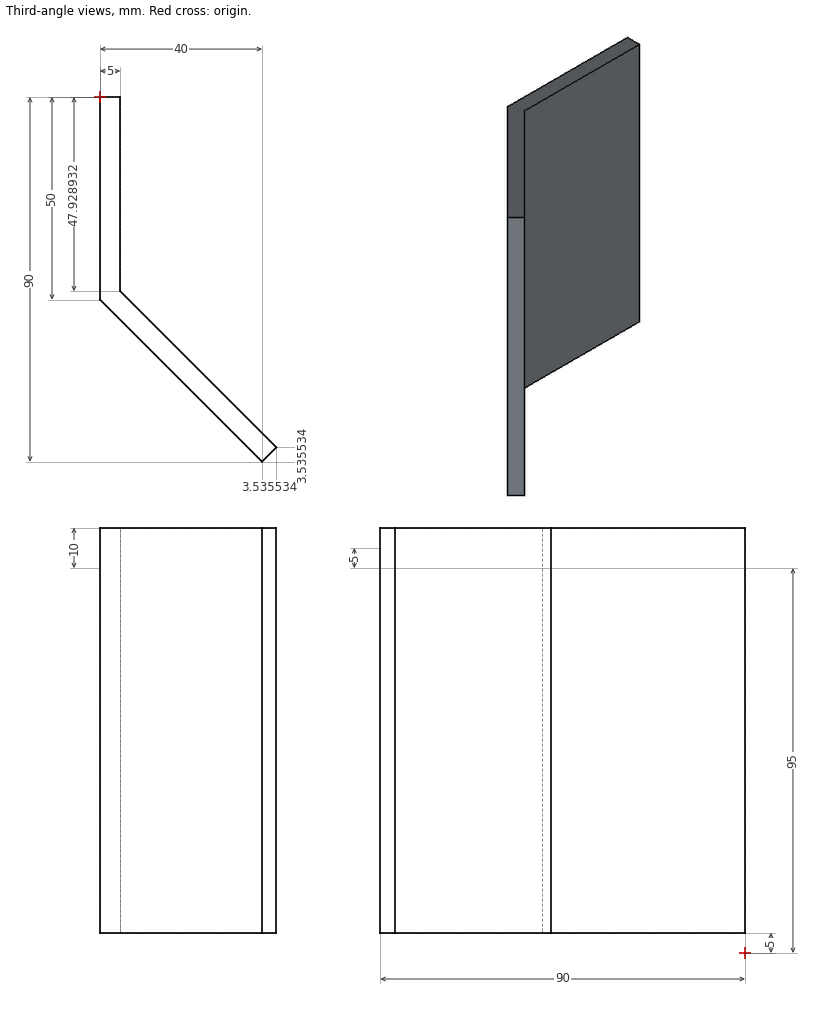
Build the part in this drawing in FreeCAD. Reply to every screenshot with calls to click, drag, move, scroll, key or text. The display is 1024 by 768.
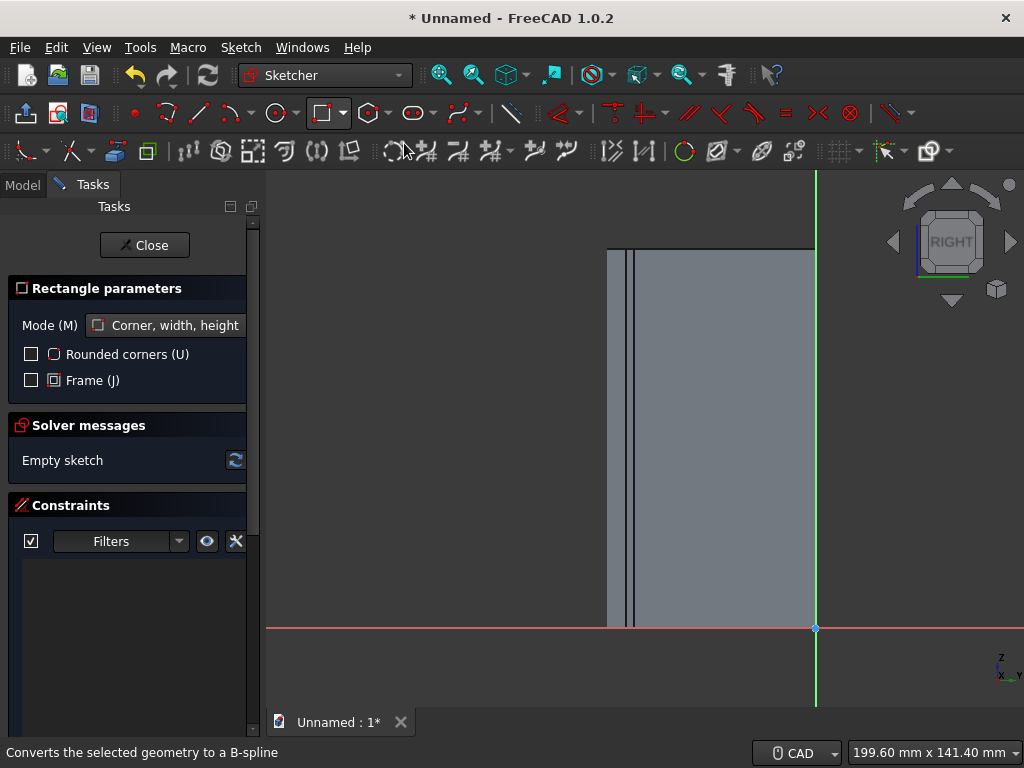
click(816, 628)
click(474, 609)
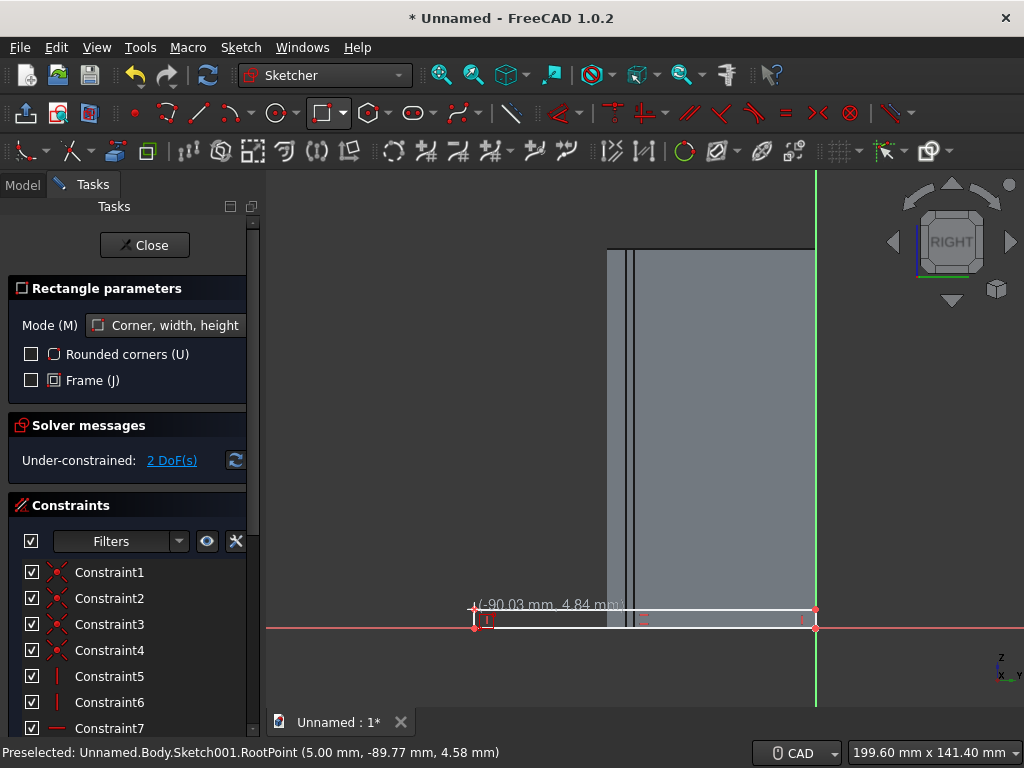
click(474, 249)
click(816, 268)
key(Escape)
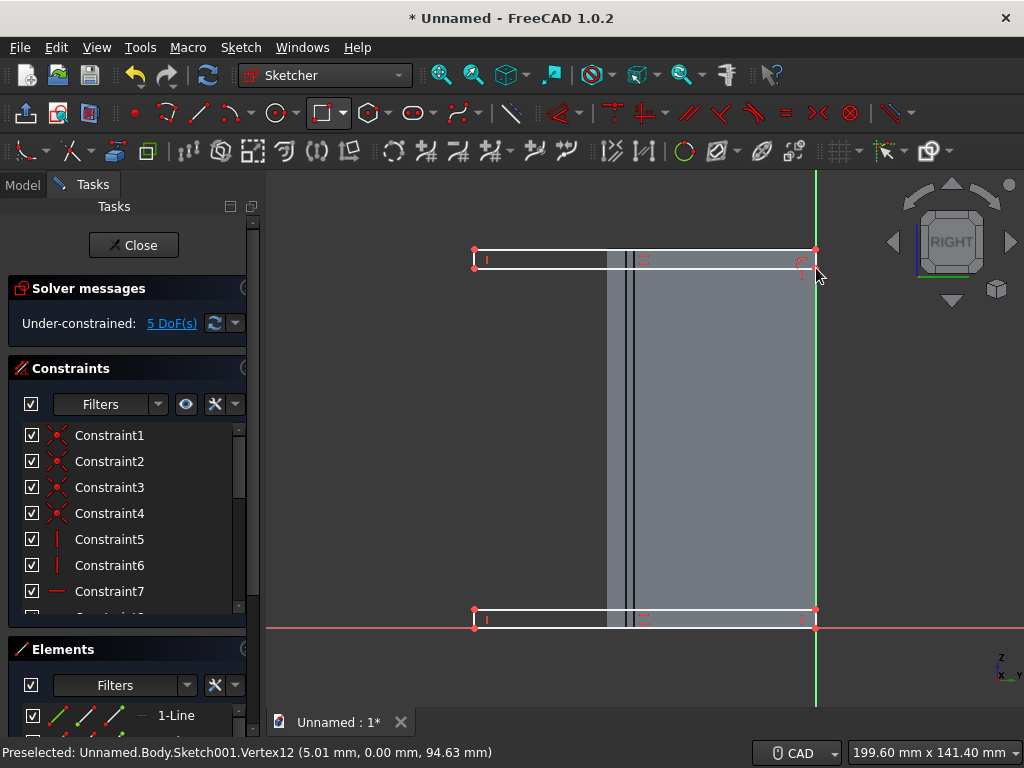
click(558, 114)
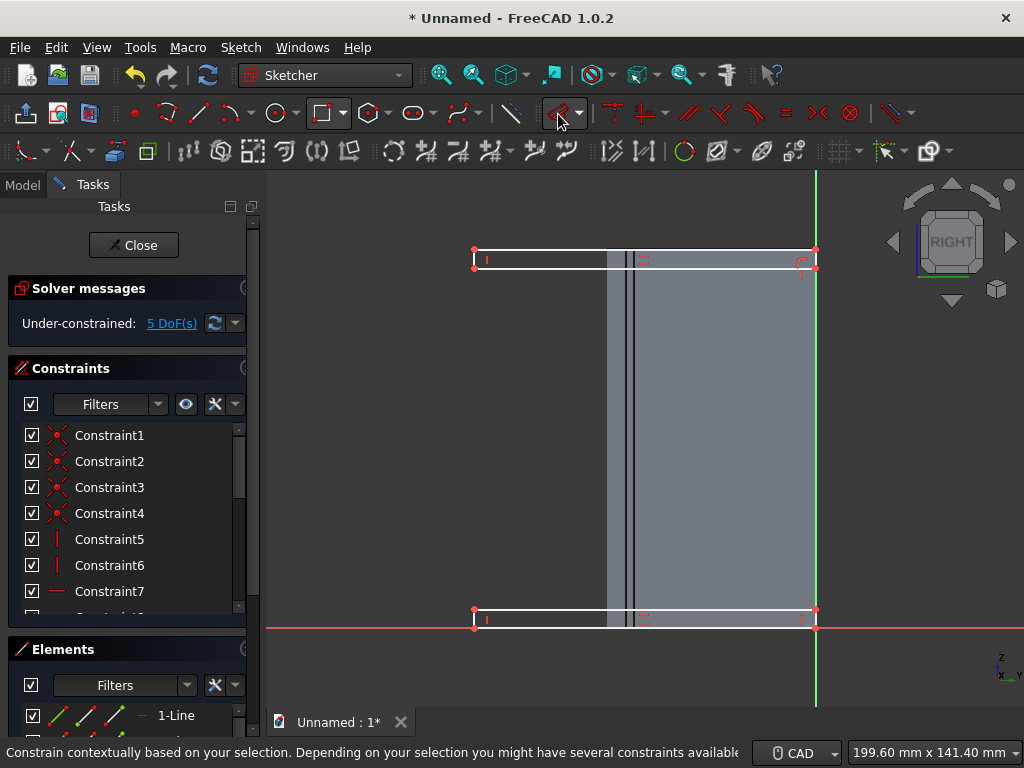
scroll(816, 619, up, 4)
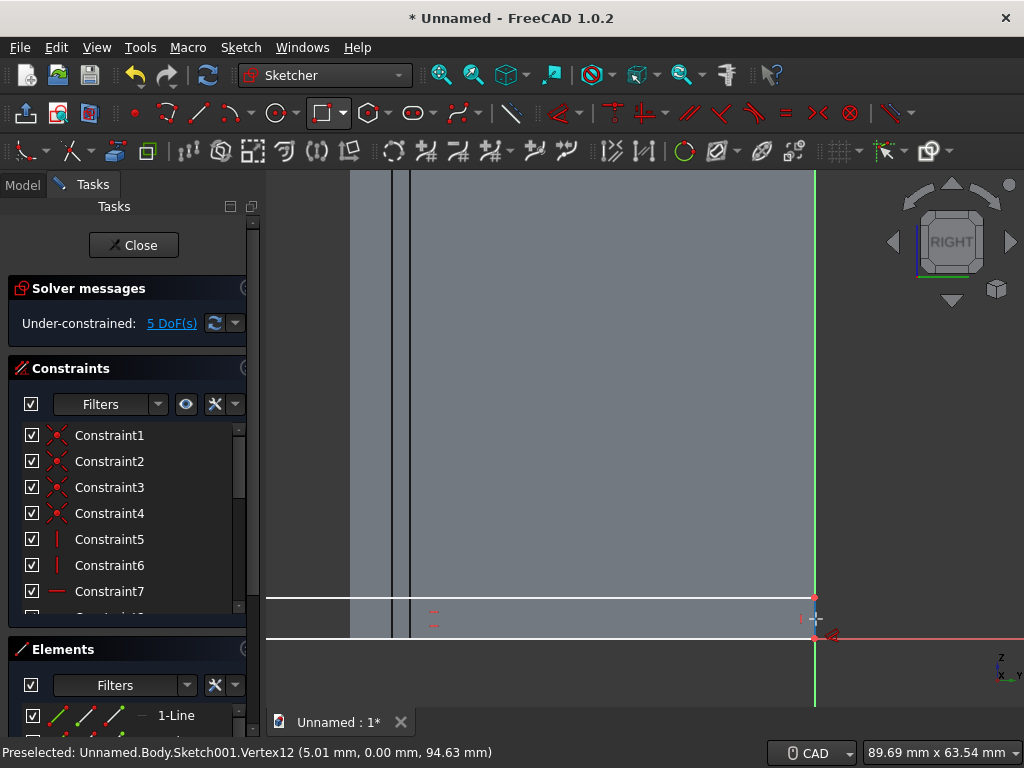
click(815, 618)
click(849, 618)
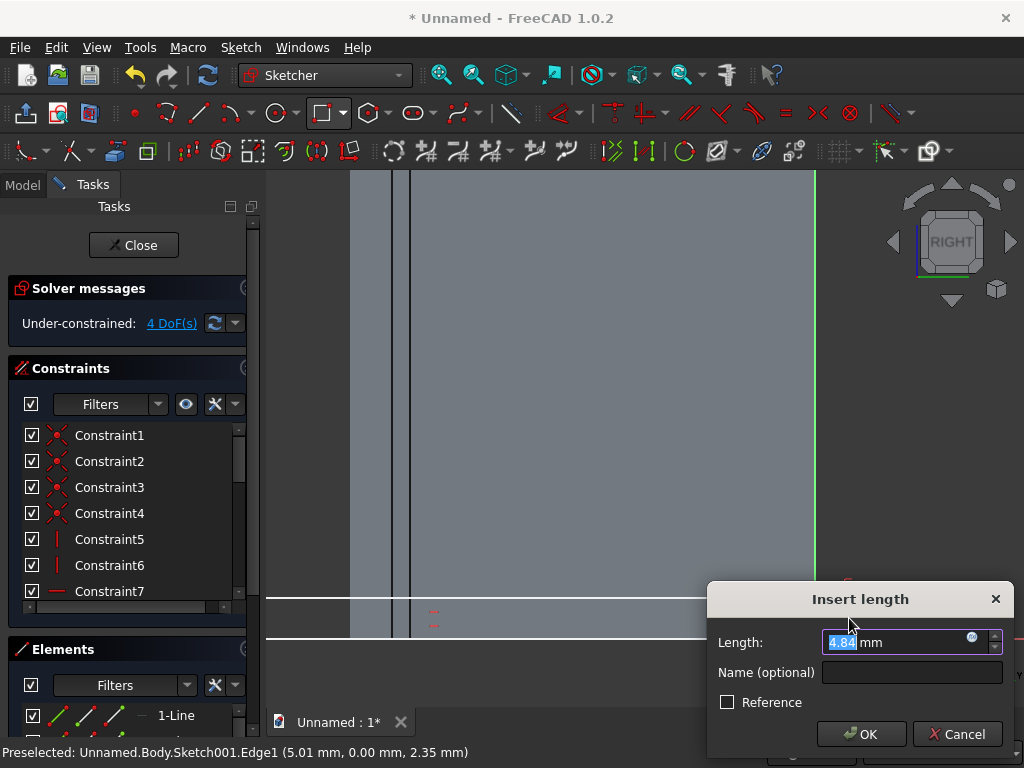
text(5)
key(Return)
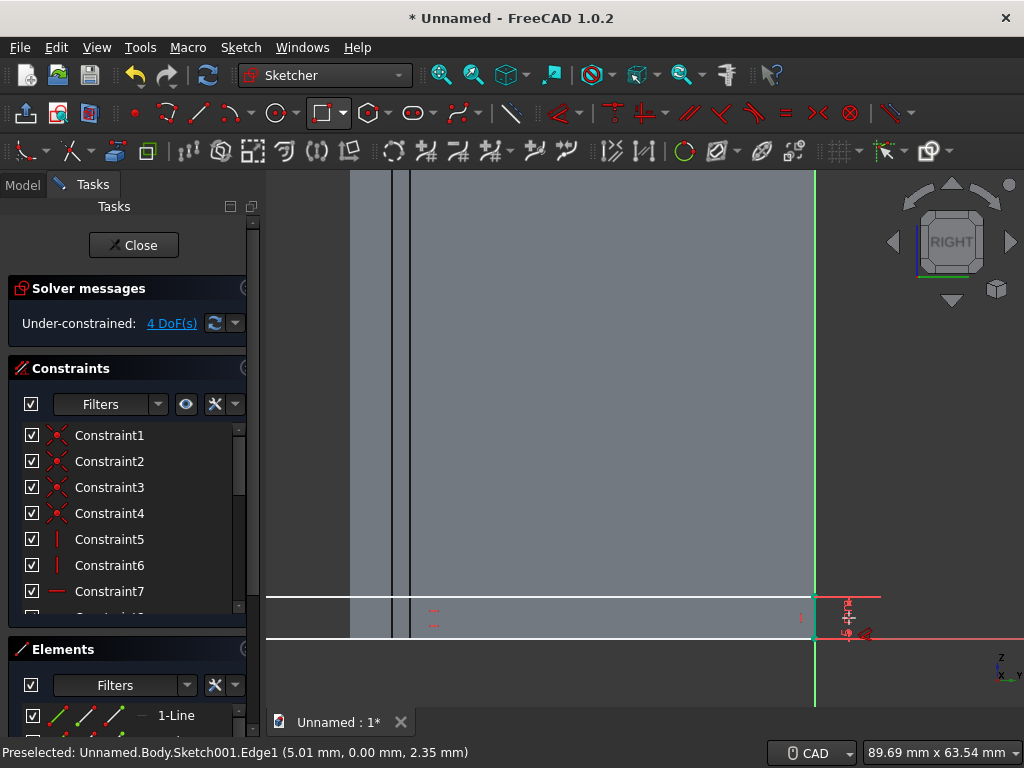
scroll(659, 568, down, 5)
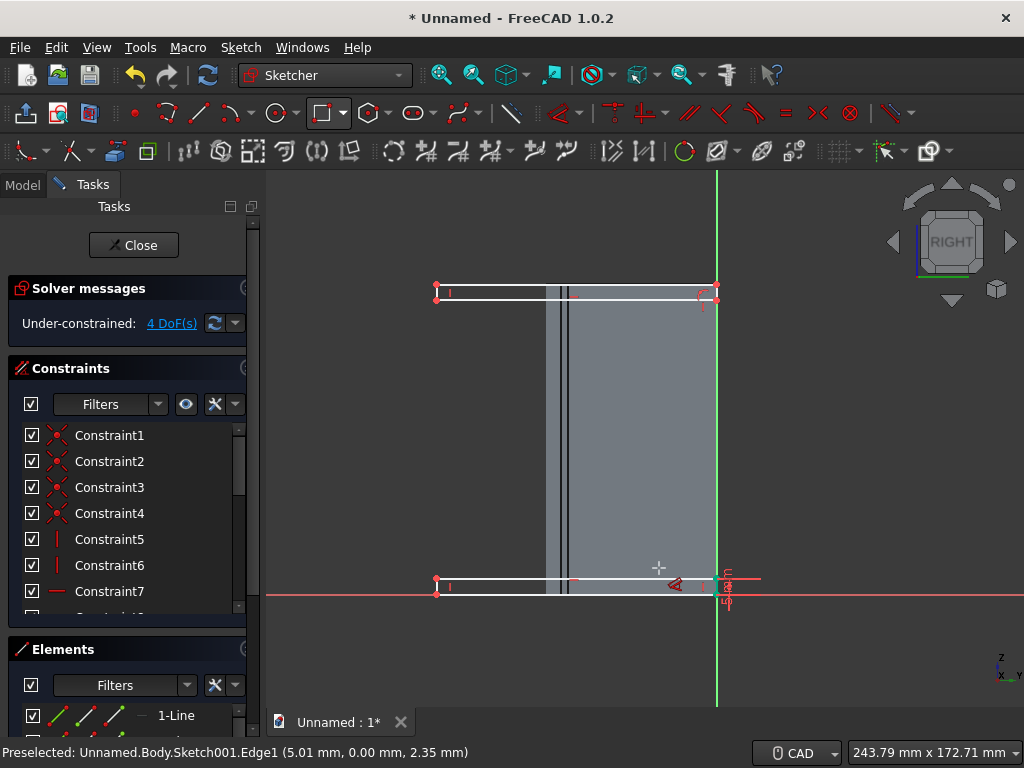
scroll(437, 289, up, 6)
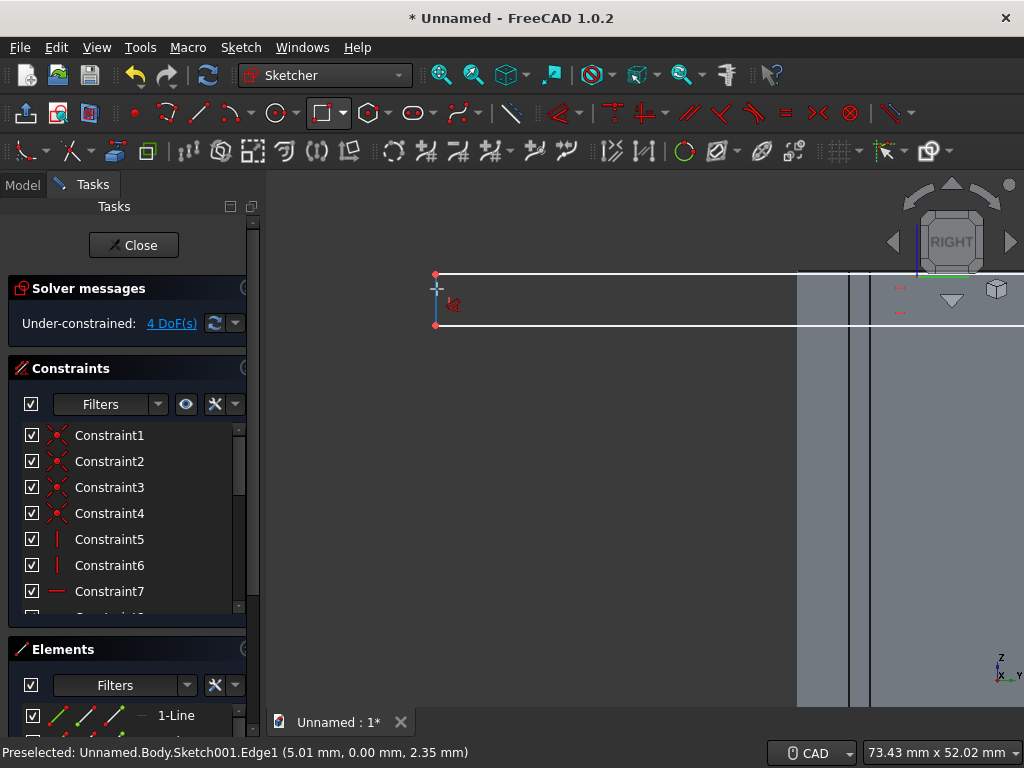
click(436, 290)
click(402, 300)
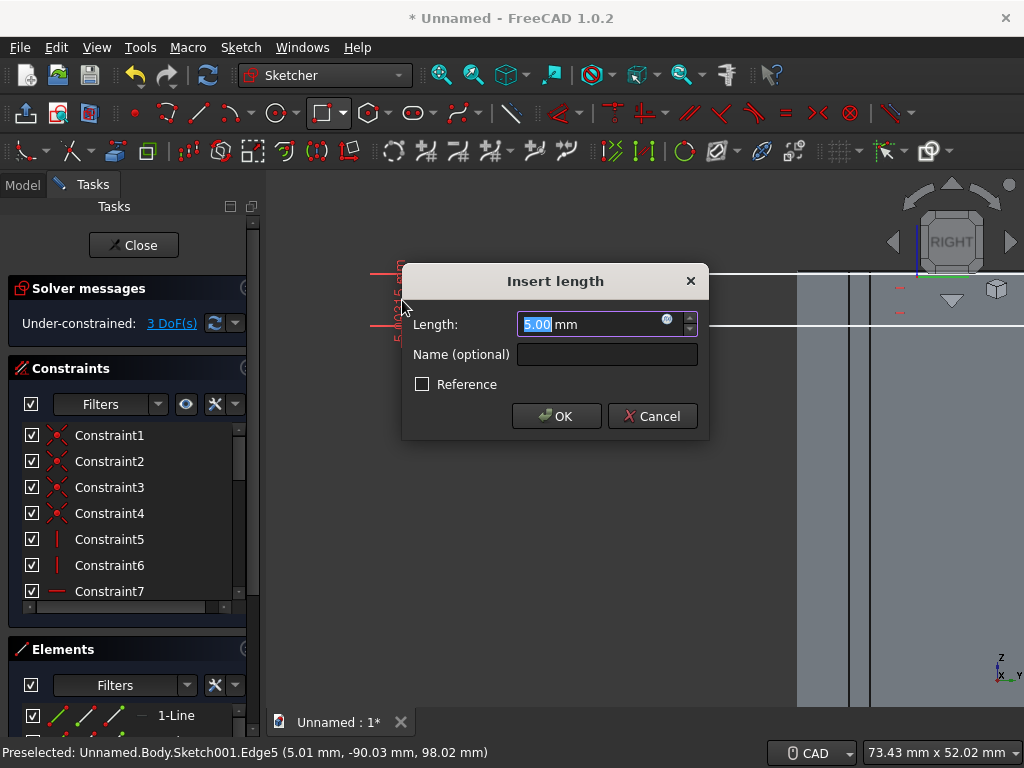
text(5)
key(Return)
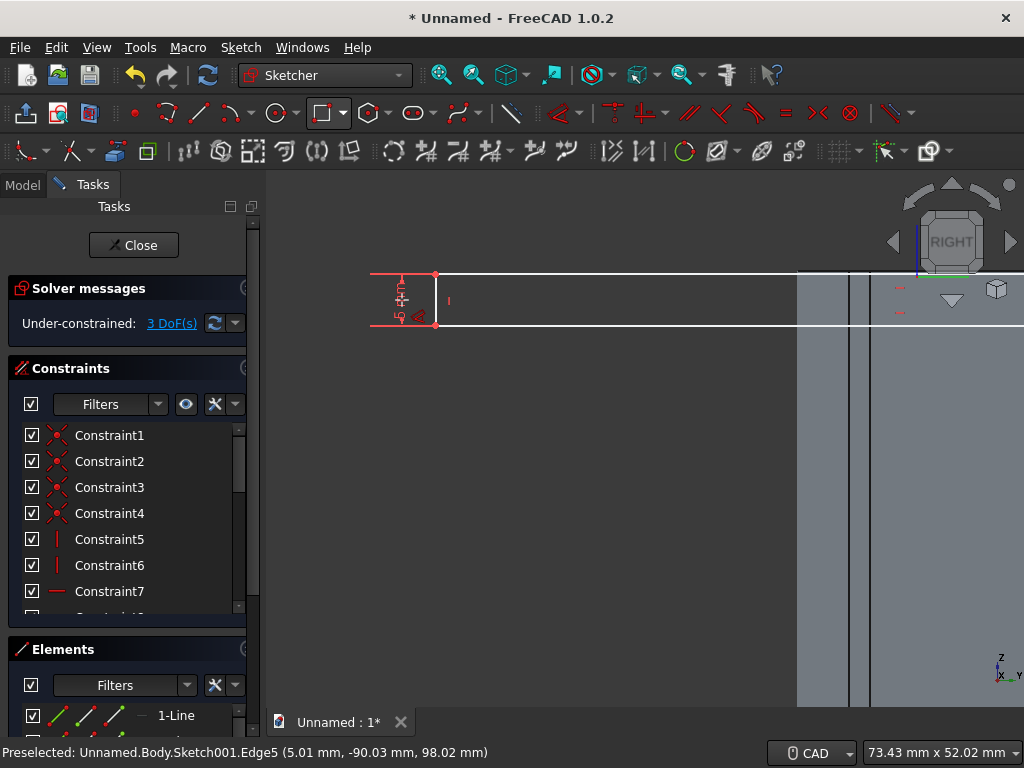
scroll(437, 288, down, 6)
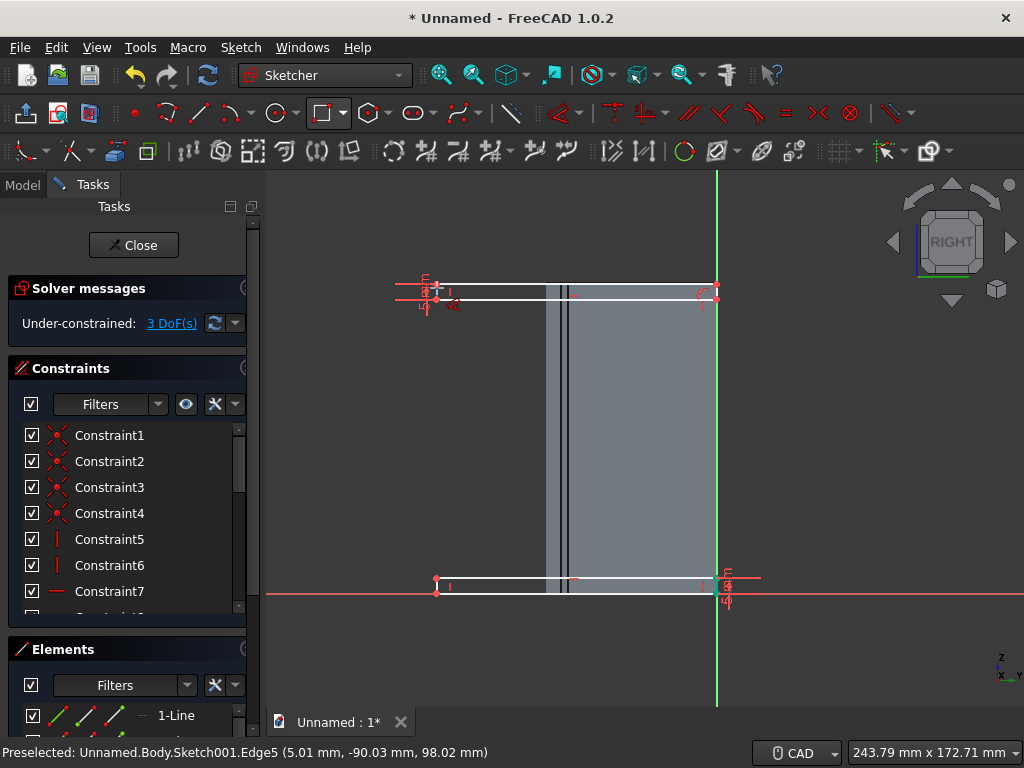
click(633, 578)
click(577, 612)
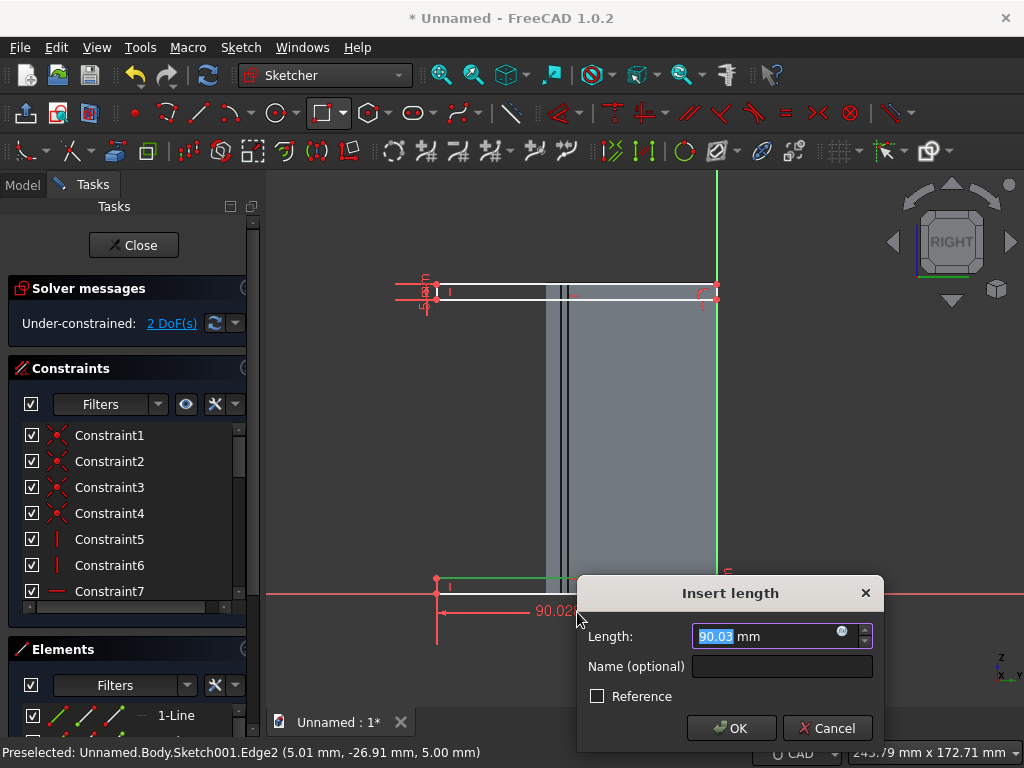
text(90)
key(Return)